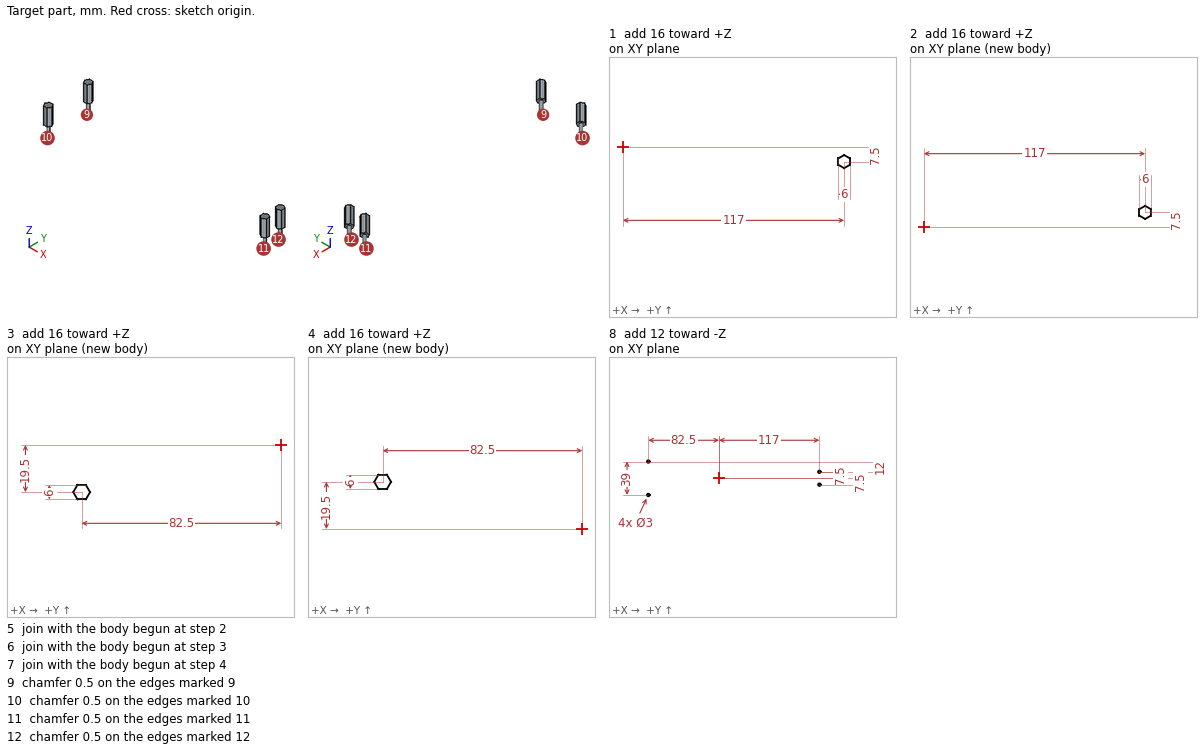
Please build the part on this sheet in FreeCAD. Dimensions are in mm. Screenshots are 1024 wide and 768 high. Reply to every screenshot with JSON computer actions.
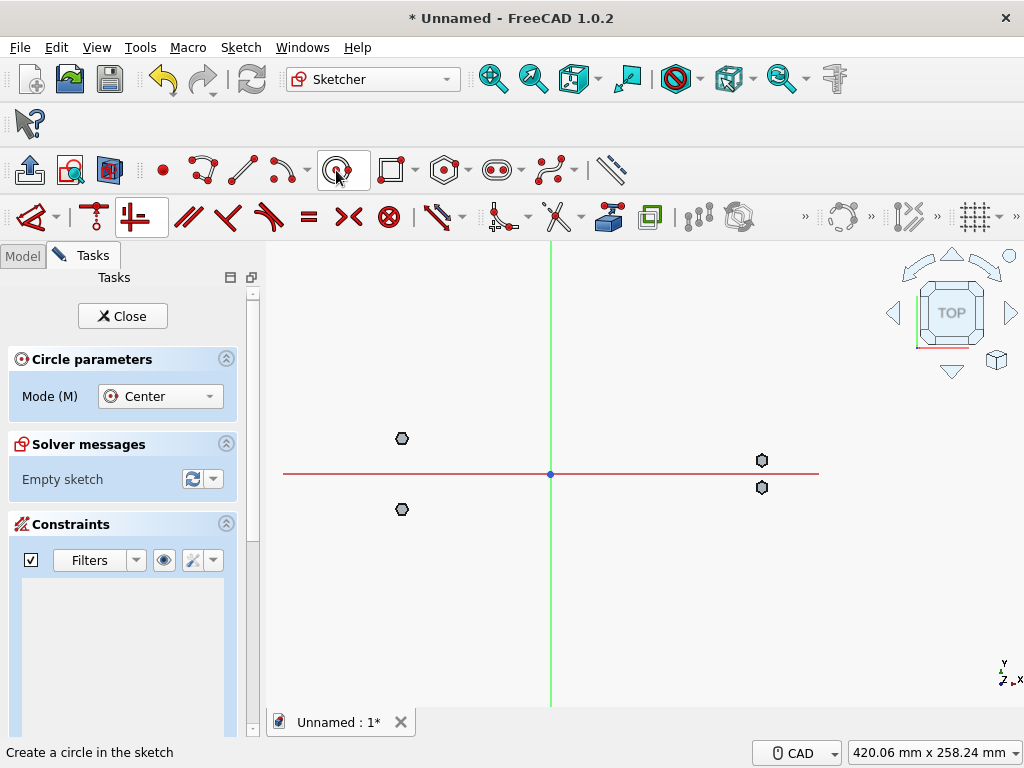
{"action": "scroll", "coordinate": [402, 439], "scroll_direction": "up", "scroll_amount": 11}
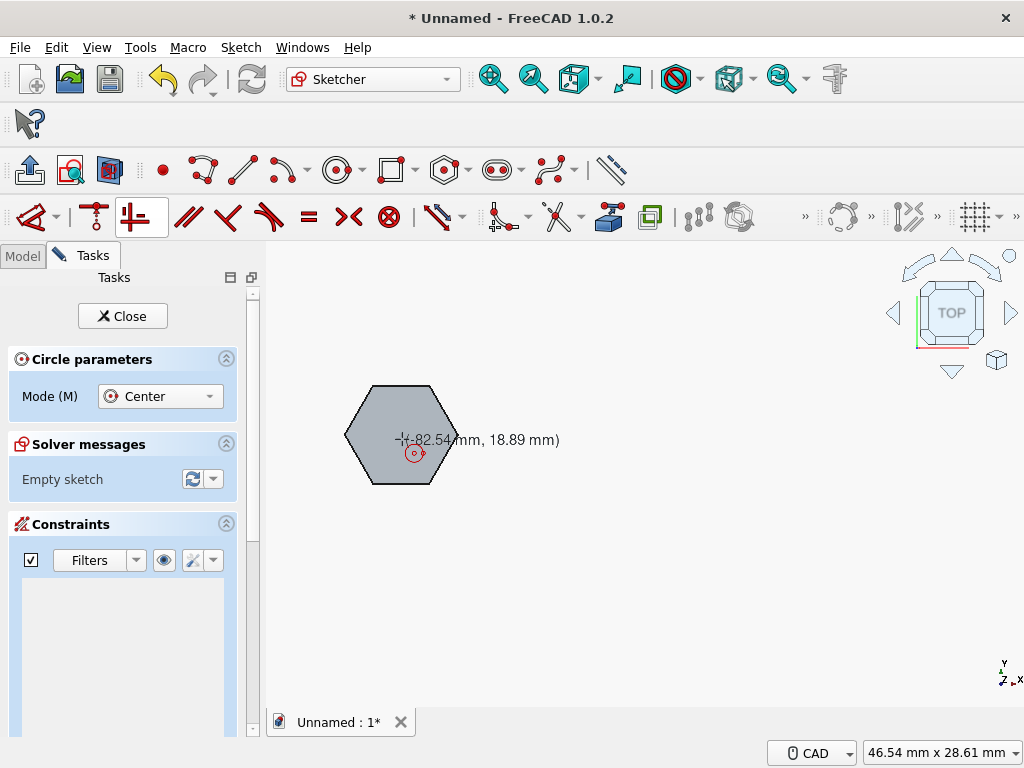
{"action": "scroll", "coordinate": [396, 439], "scroll_direction": "down", "scroll_amount": 11}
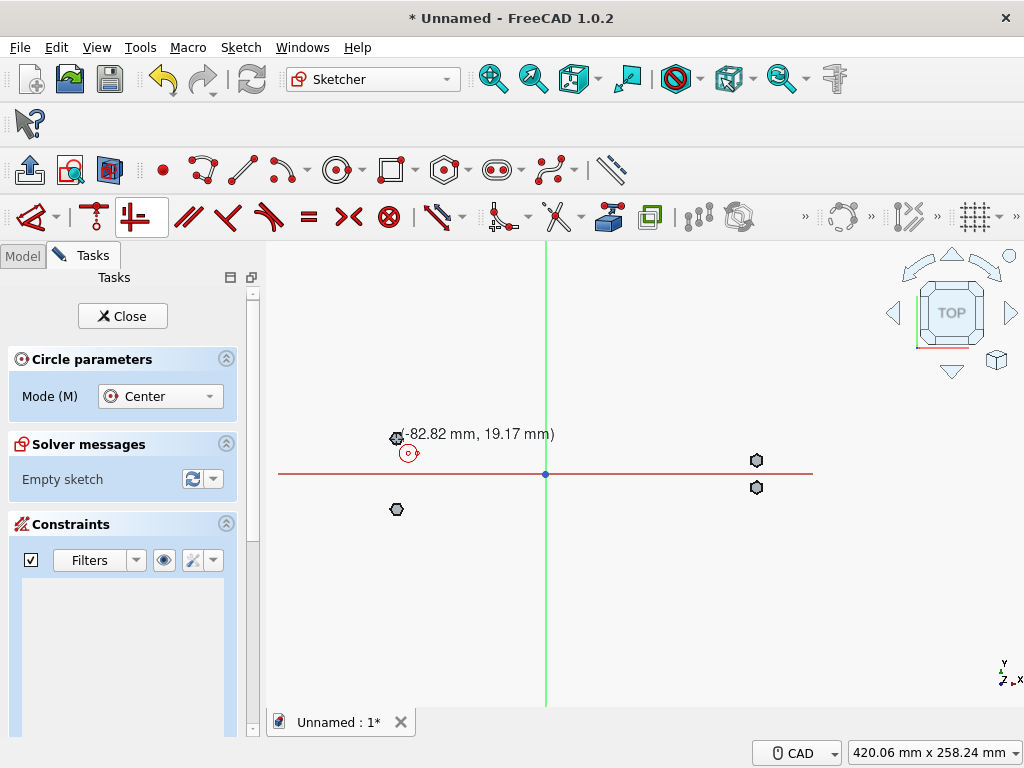
{"action": "left_click", "coordinate": [397, 439]}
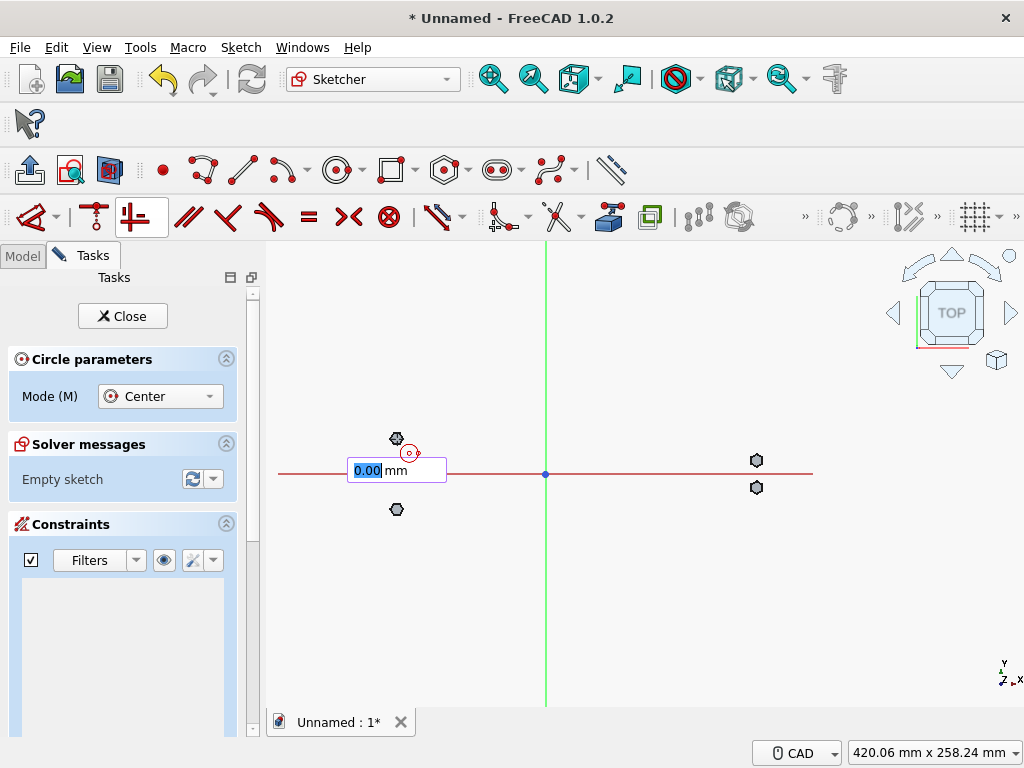
{"action": "scroll", "coordinate": [399, 437], "scroll_direction": "up", "scroll_amount": 9}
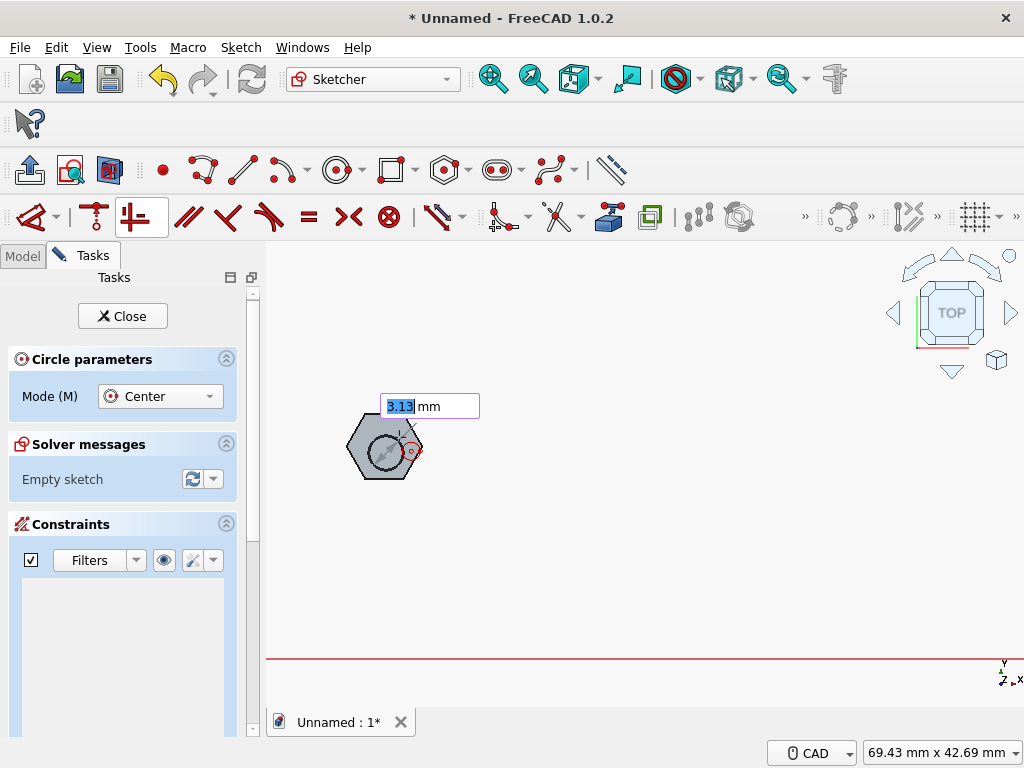
{"action": "left_click", "coordinate": [396, 435]}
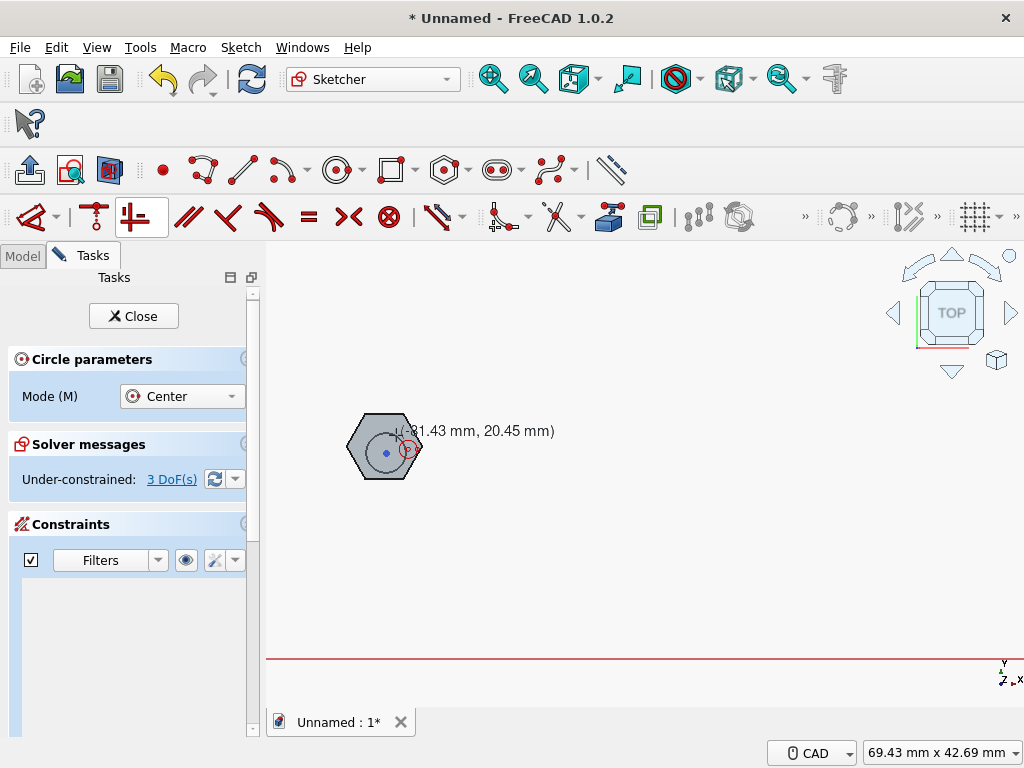
{"action": "scroll", "coordinate": [399, 437], "scroll_direction": "down", "scroll_amount": 9}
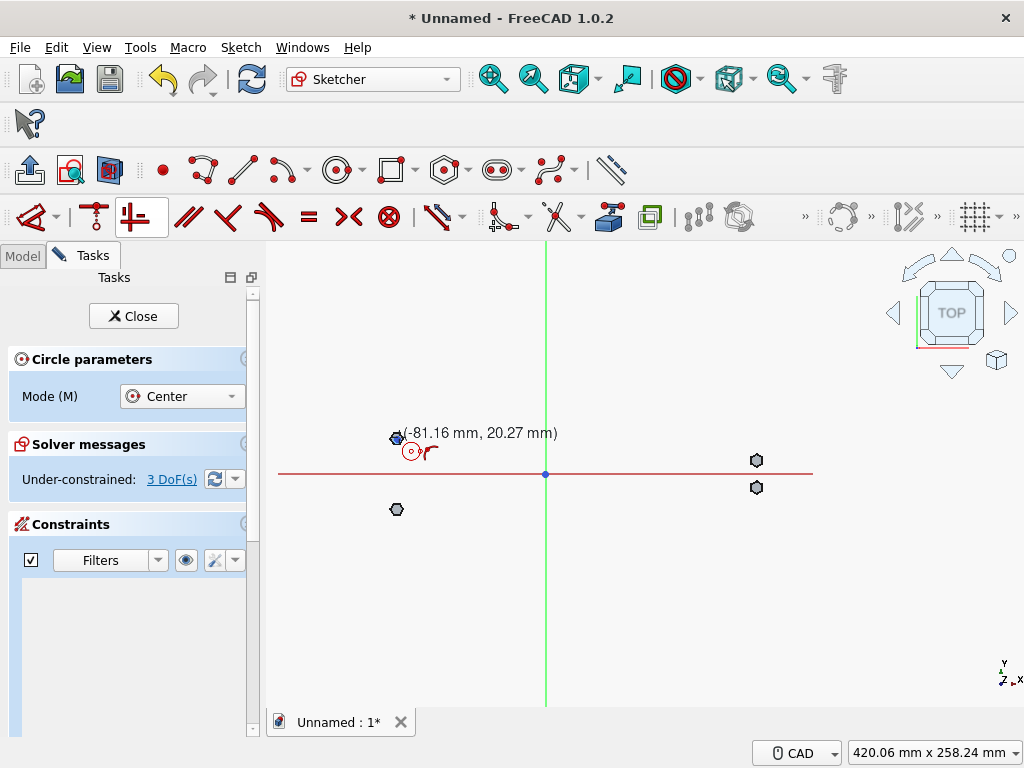
{"action": "scroll", "coordinate": [397, 509], "scroll_direction": "up", "scroll_amount": 11}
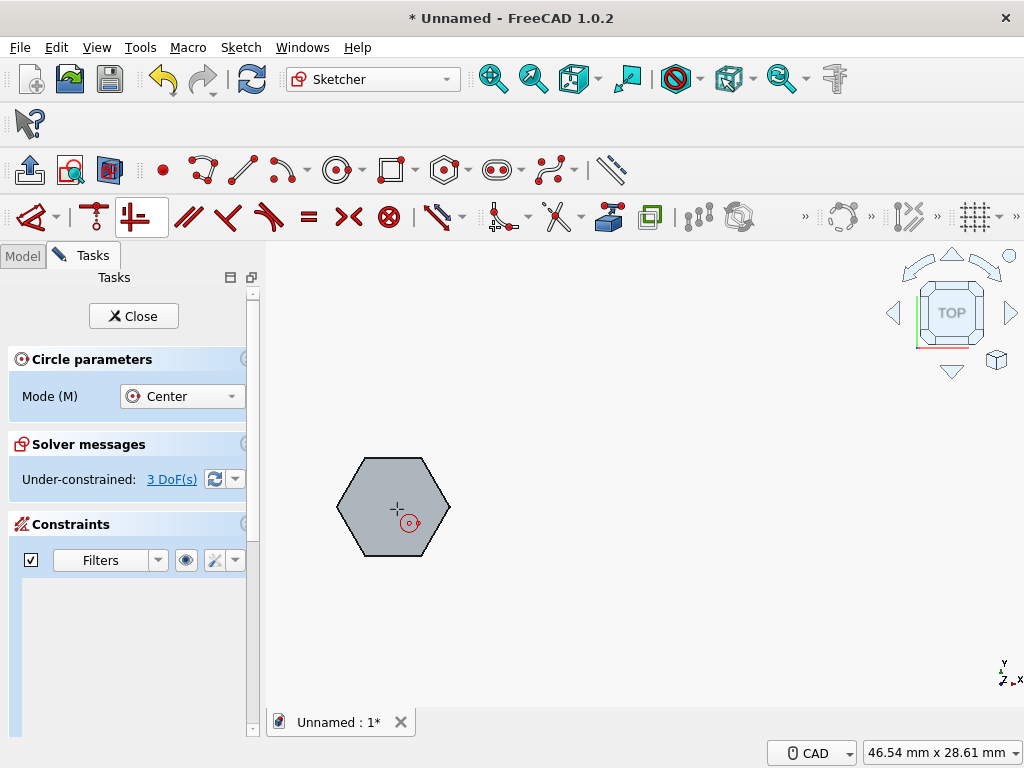
{"action": "scroll", "coordinate": [397, 509], "scroll_direction": "down", "scroll_amount": 11}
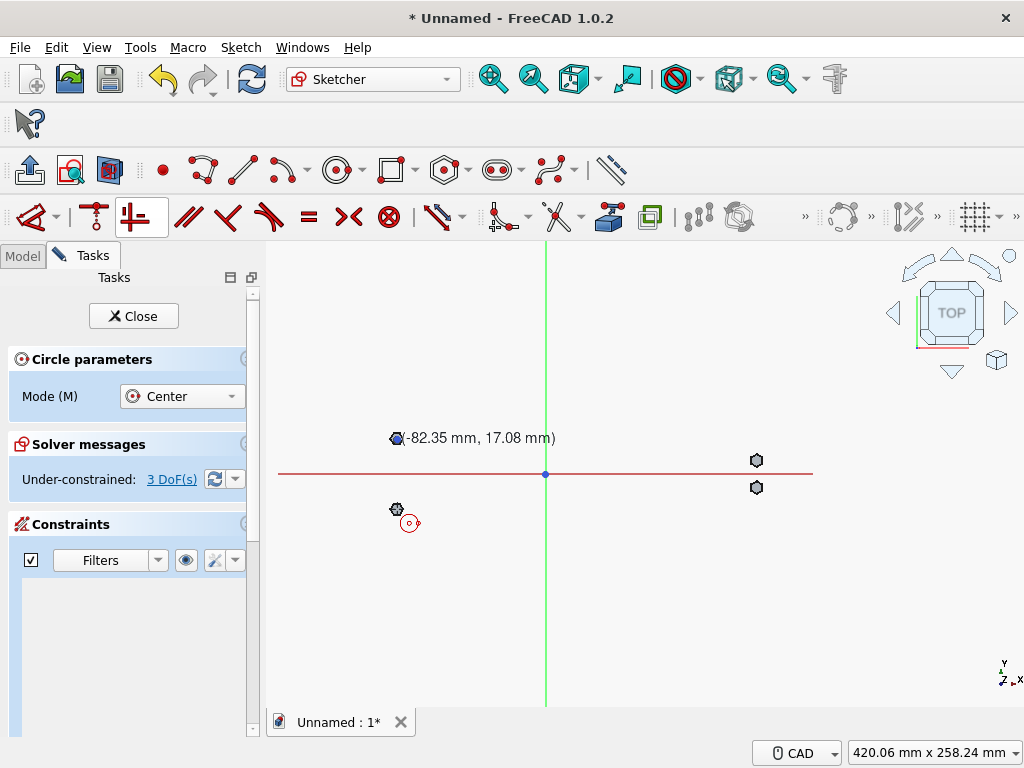
{"action": "left_click", "coordinate": [397, 509]}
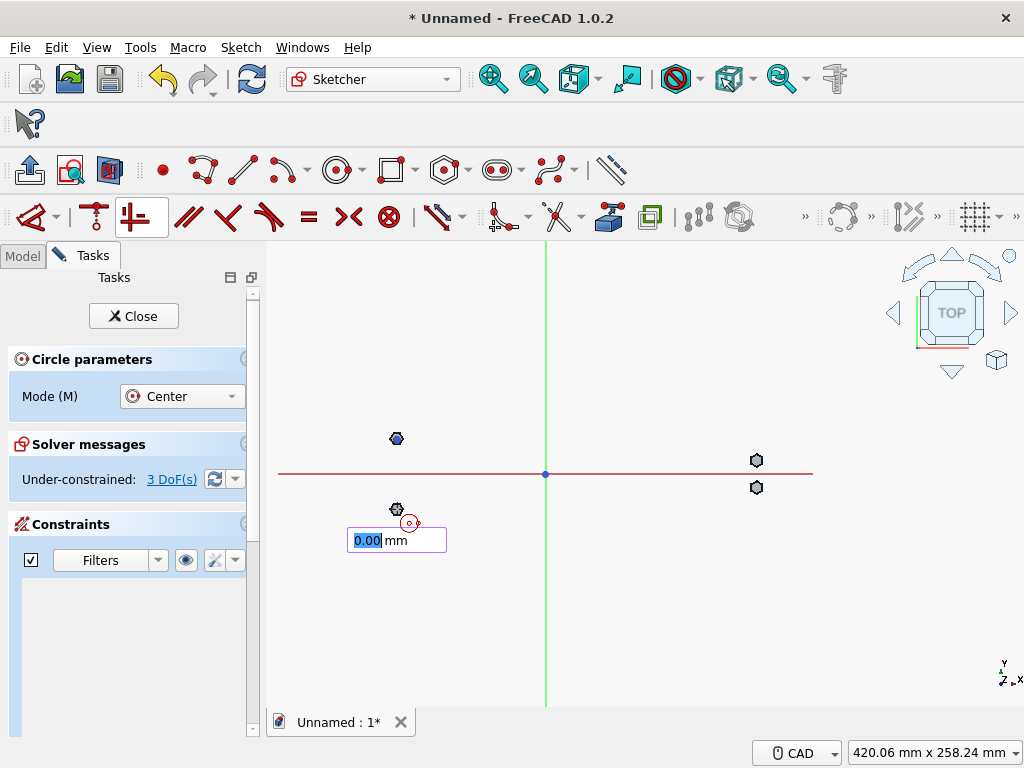
{"action": "scroll", "coordinate": [399, 507], "scroll_direction": "up", "scroll_amount": 9}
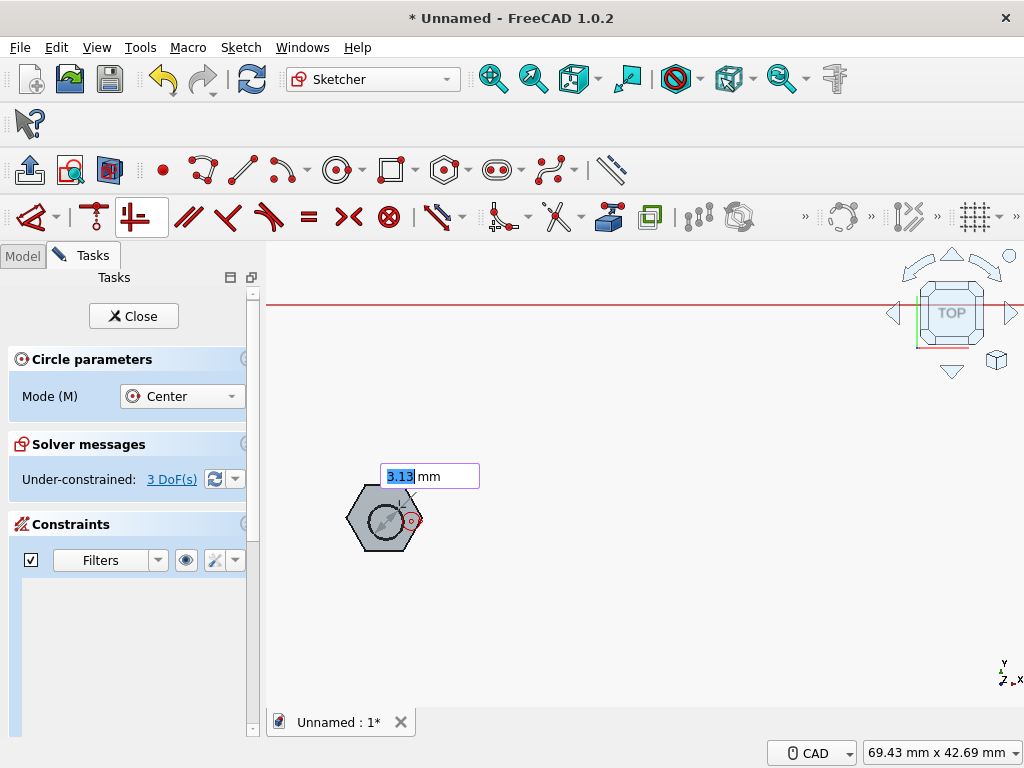
{"action": "left_click", "coordinate": [396, 506]}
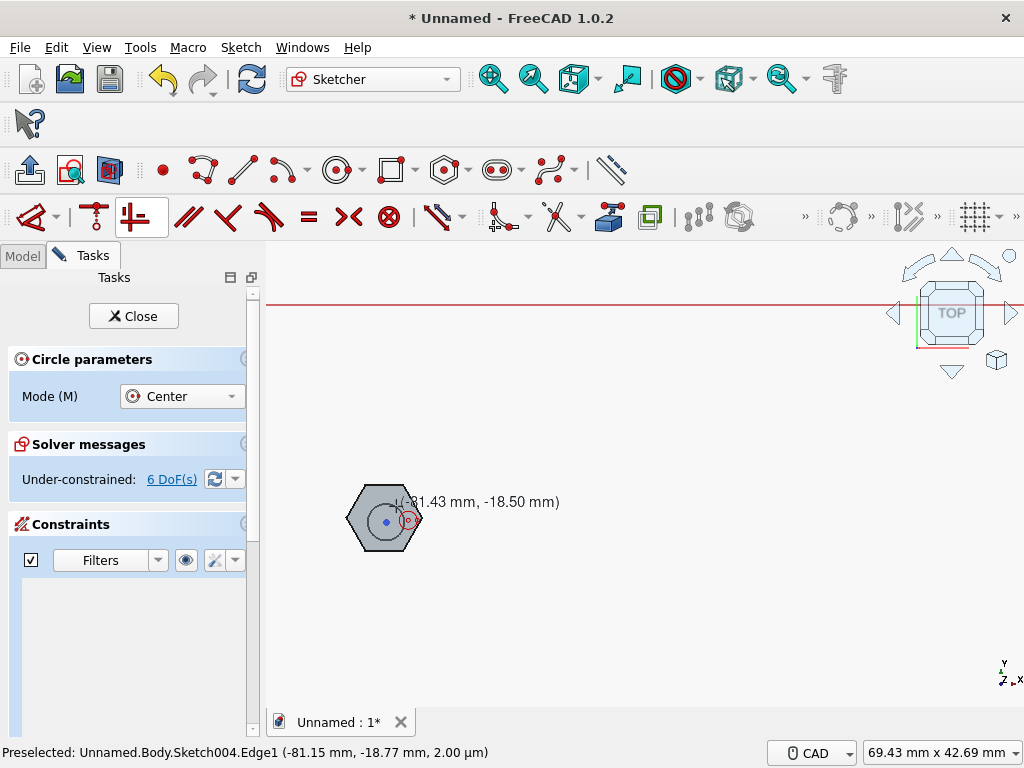
{"action": "scroll", "coordinate": [399, 507], "scroll_direction": "down", "scroll_amount": 9}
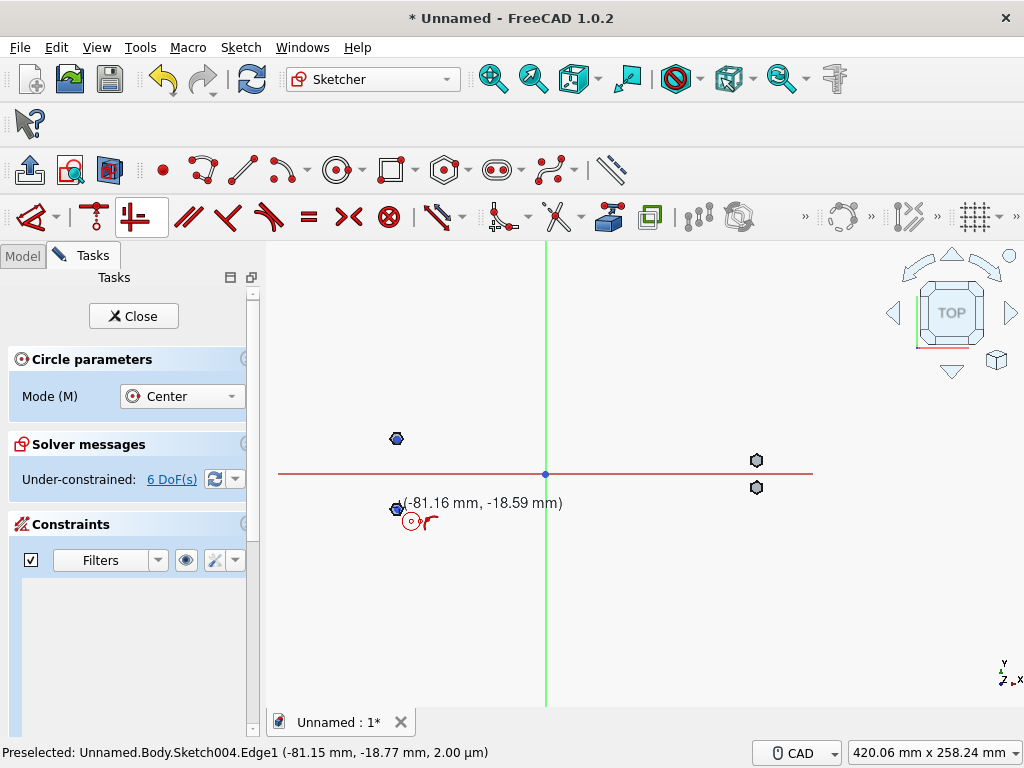
{"action": "scroll", "coordinate": [757, 461], "scroll_direction": "up", "scroll_amount": 11}